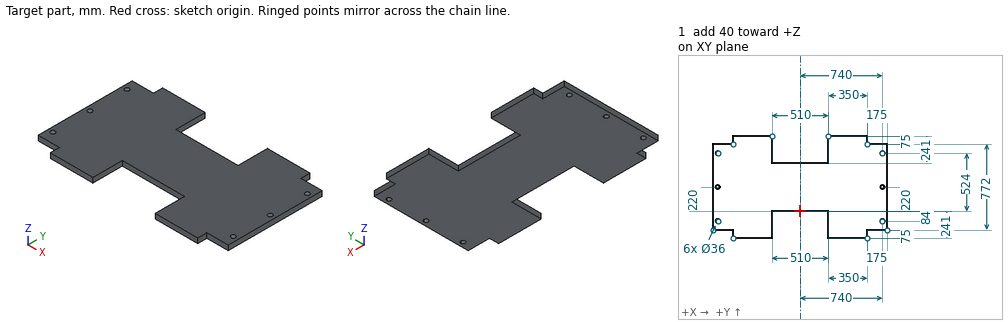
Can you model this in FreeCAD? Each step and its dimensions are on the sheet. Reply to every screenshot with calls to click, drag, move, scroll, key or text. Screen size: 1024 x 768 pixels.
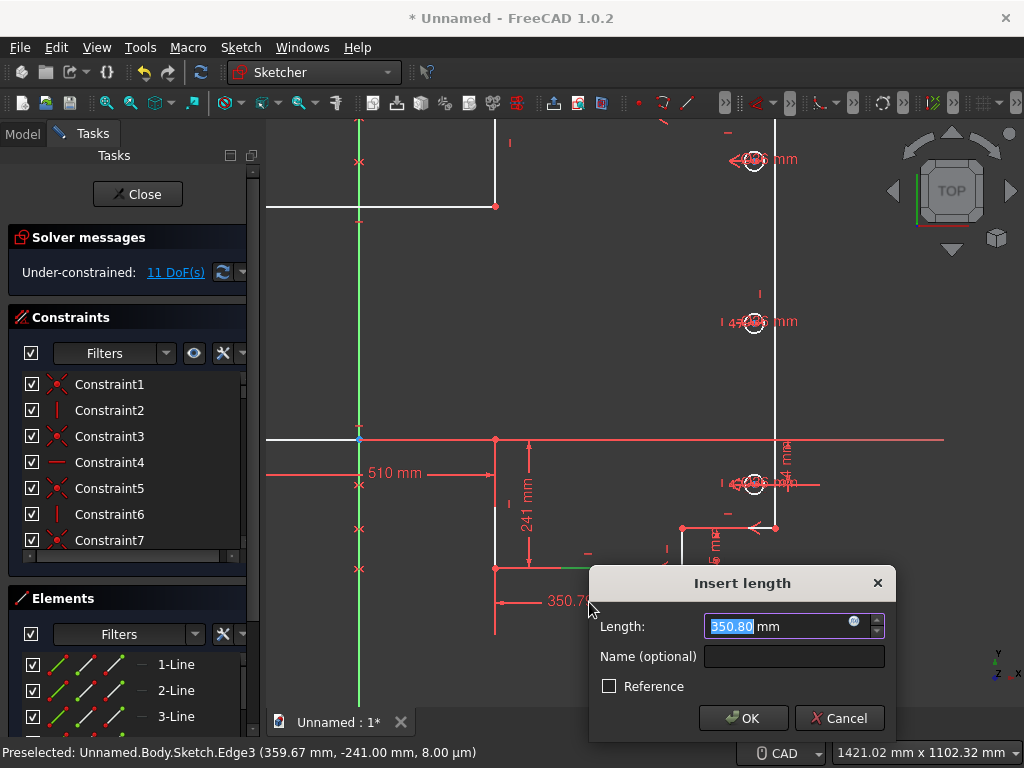
text(350)
key(Return)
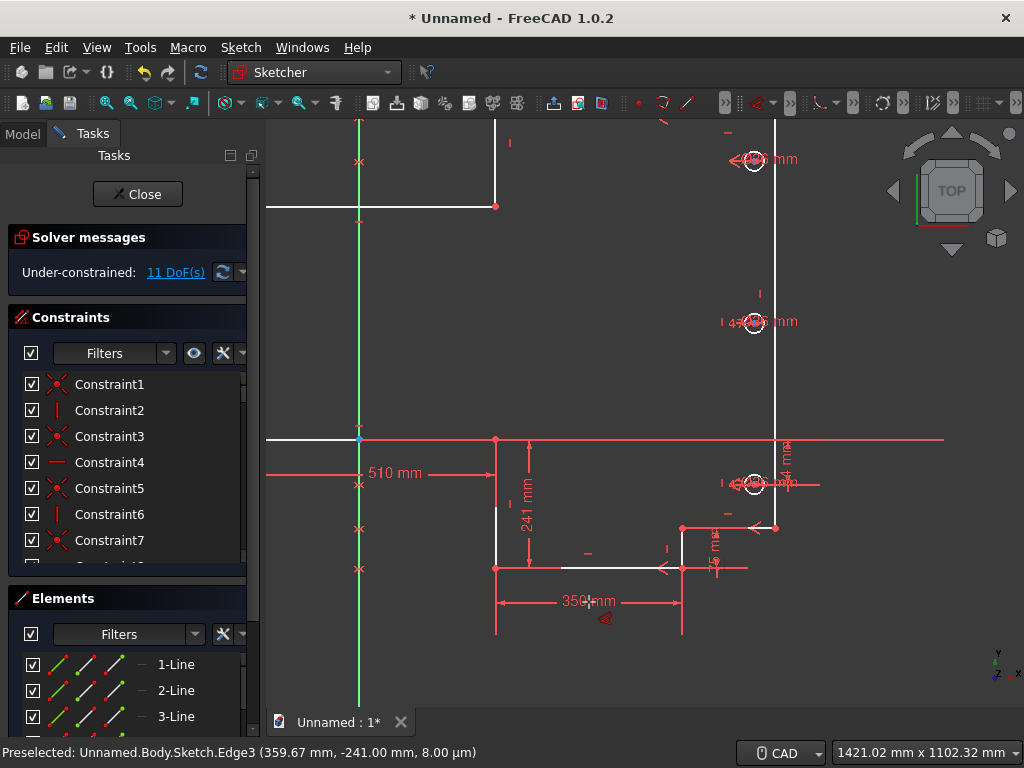
click(710, 528)
click(729, 494)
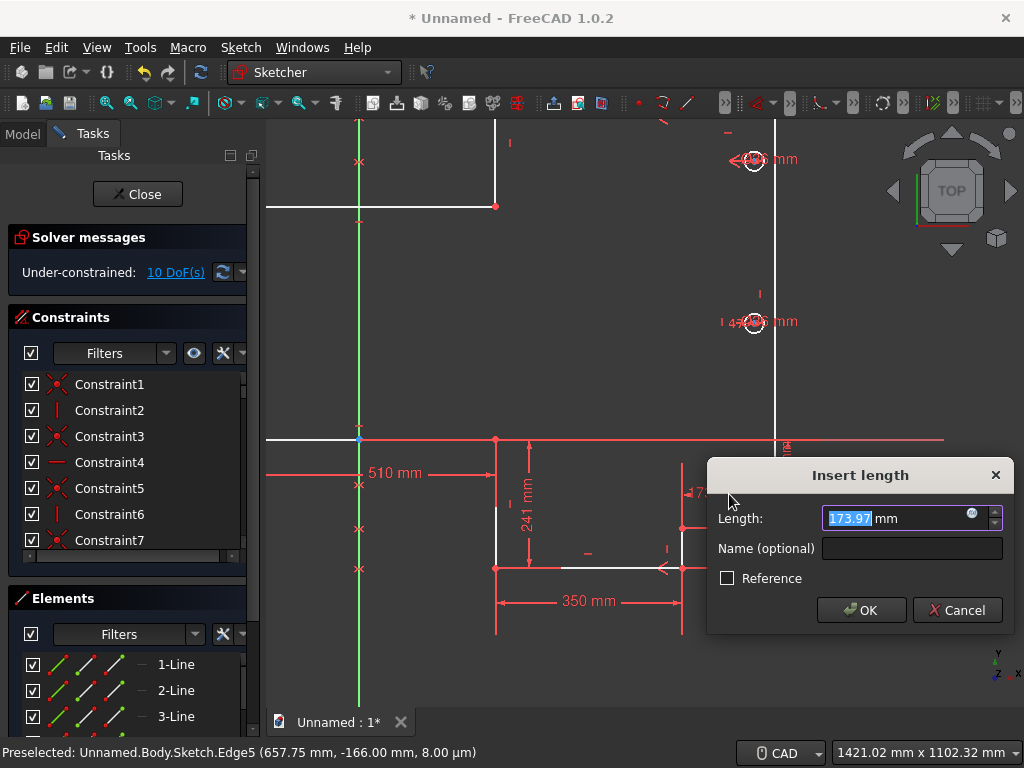
text(175)
key(Return)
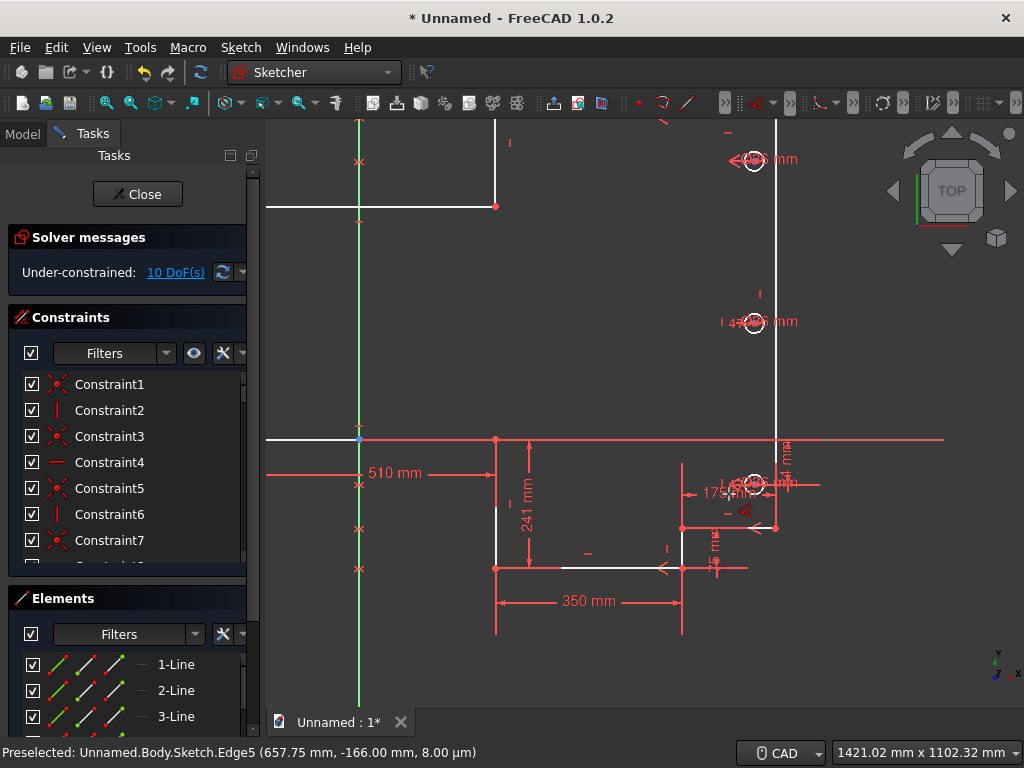
click(776, 405)
click(810, 338)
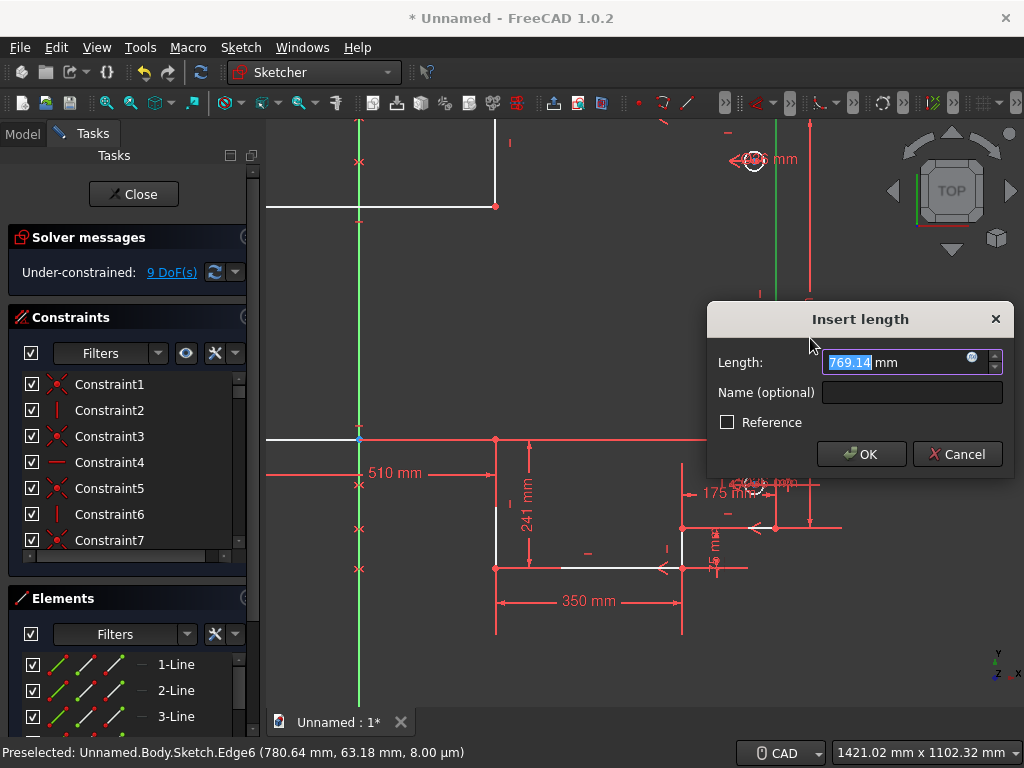
text(772)
key(Return)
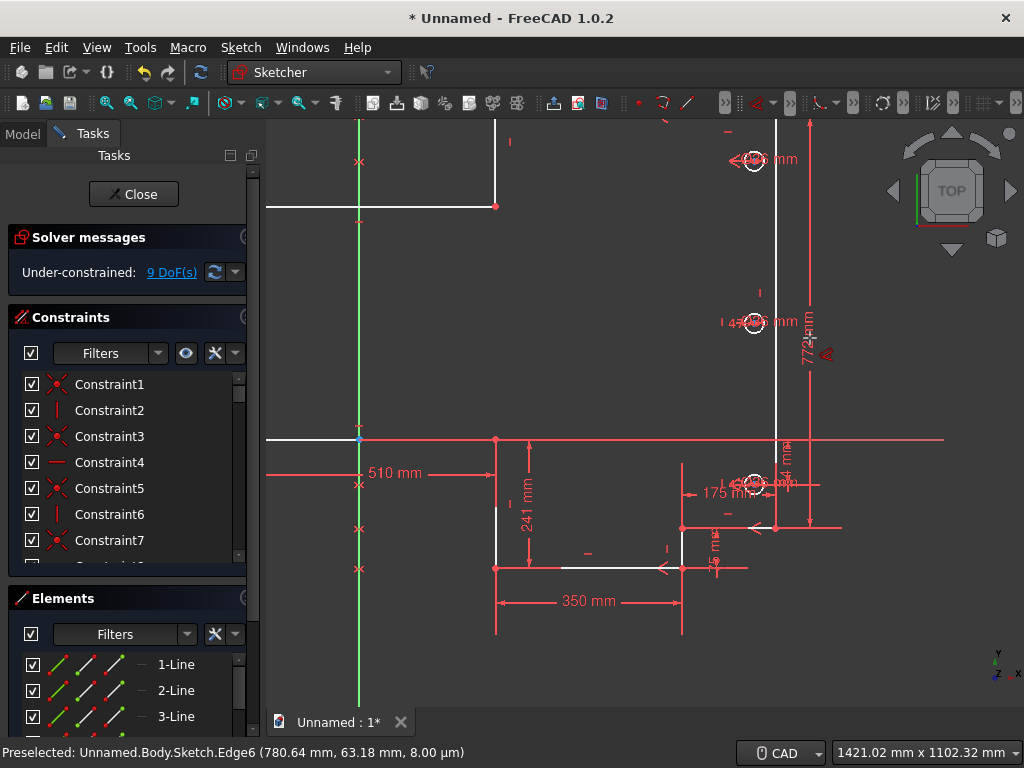
scroll(754, 487, down, 4)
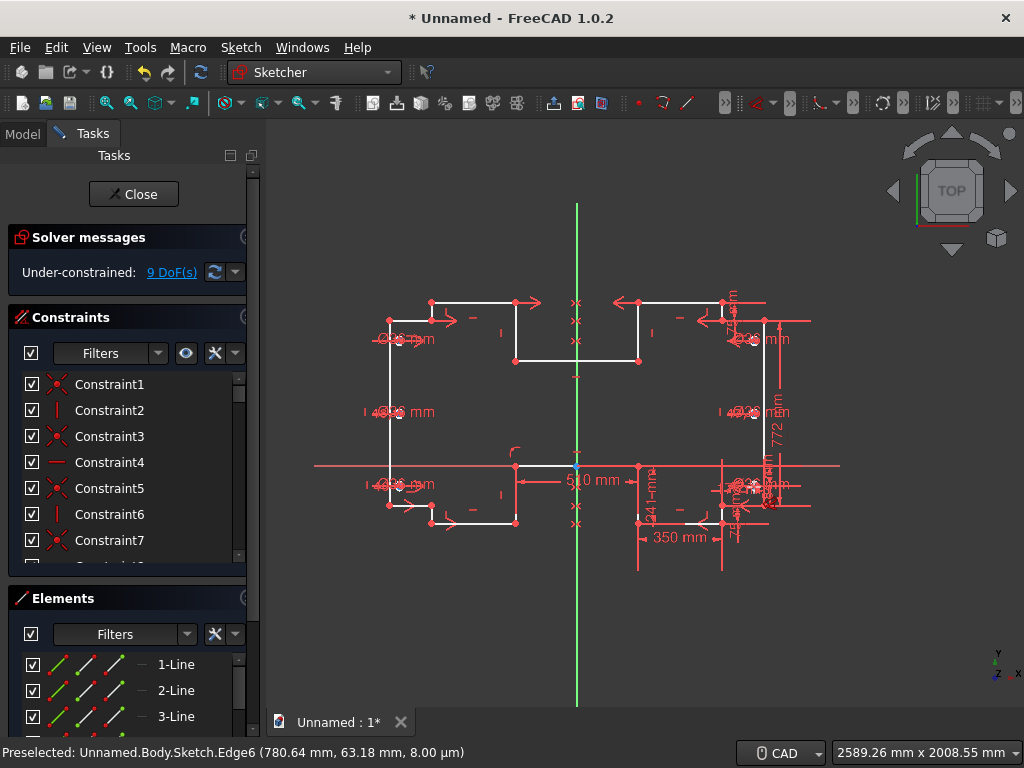
click(751, 321)
click(743, 287)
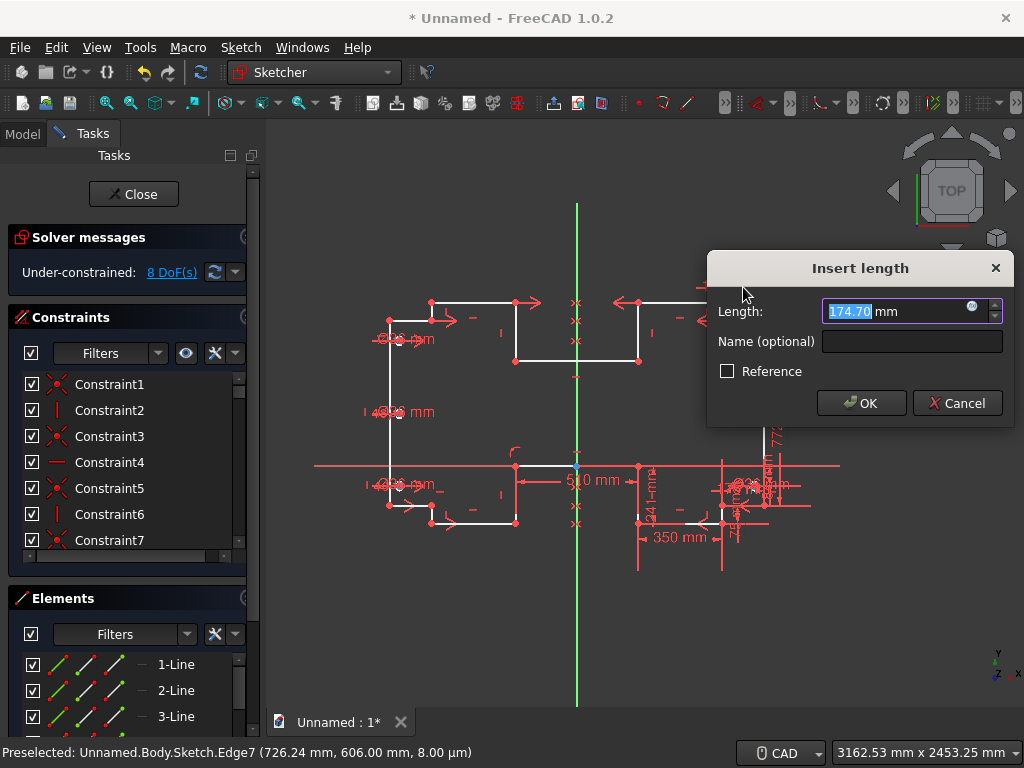
text(175)
key(Return)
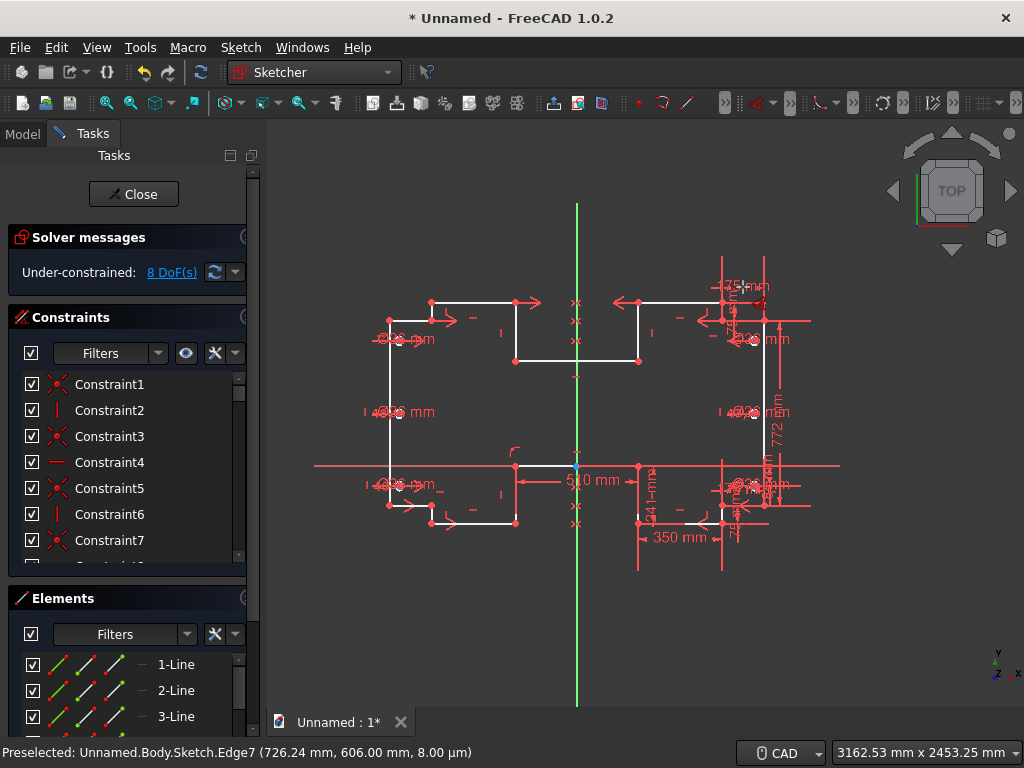
click(697, 303)
click(661, 269)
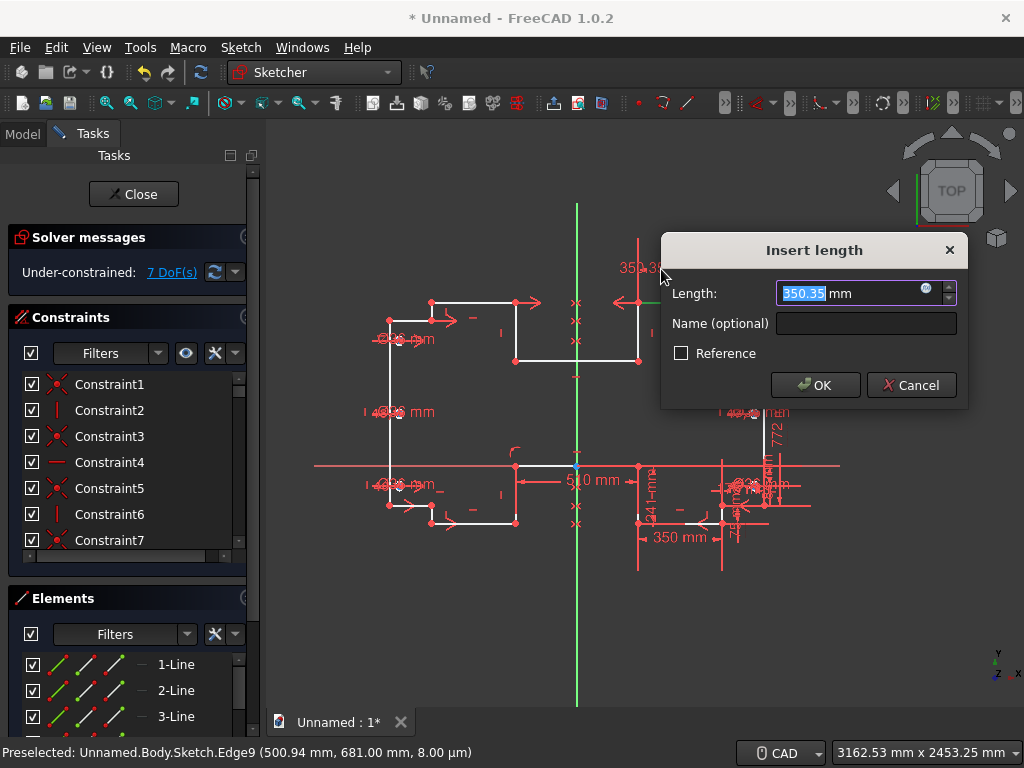
text(350)
key(Return)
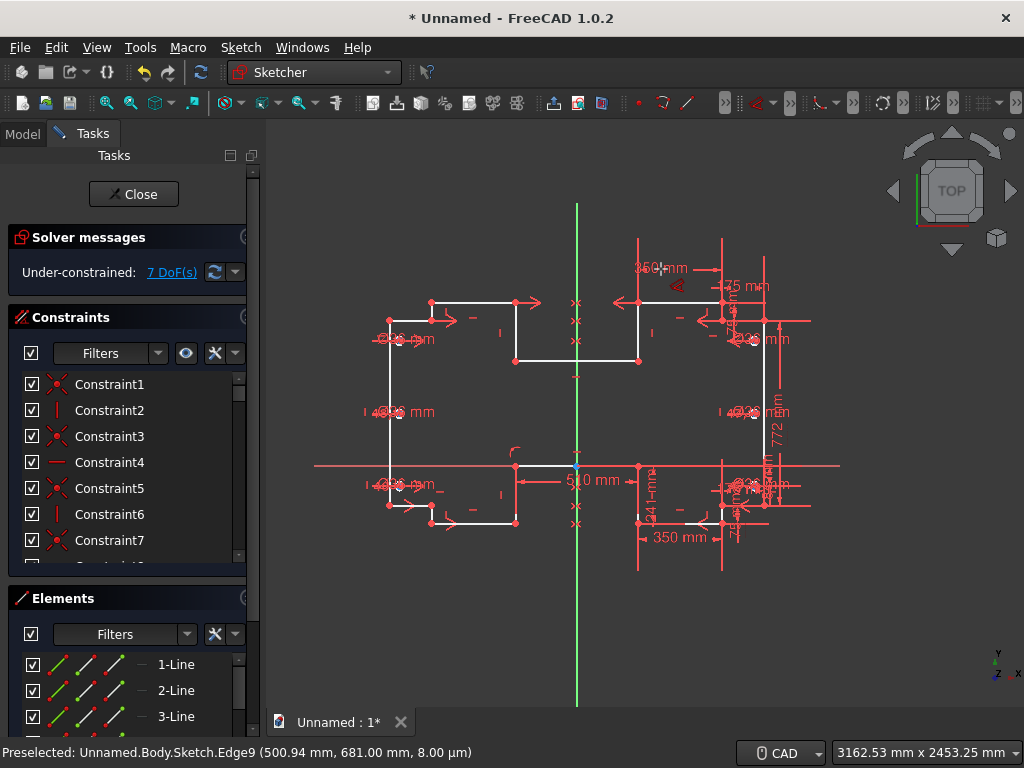
click(638, 320)
click(672, 346)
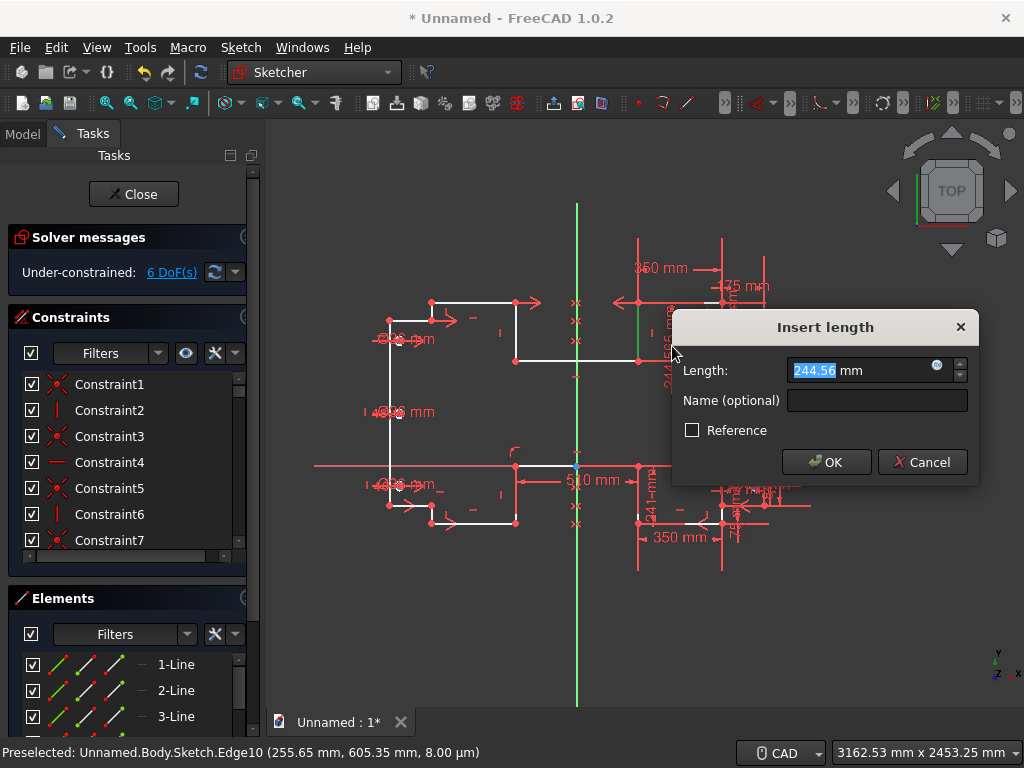
text(241)
key(Return)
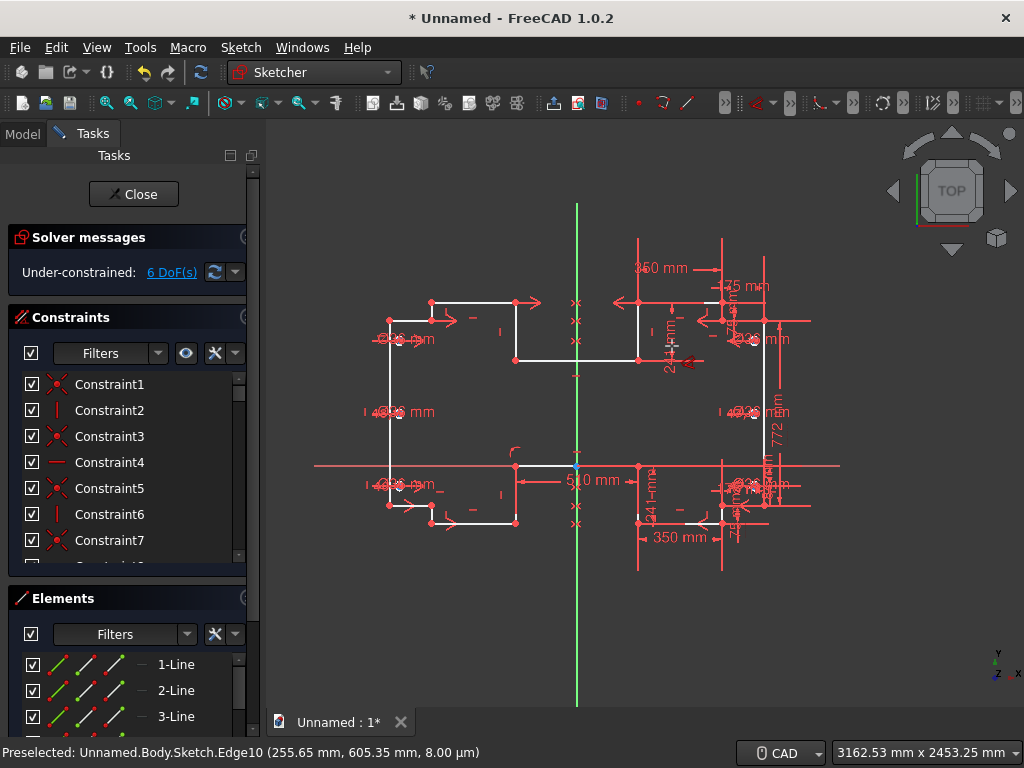
click(601, 361)
click(549, 327)